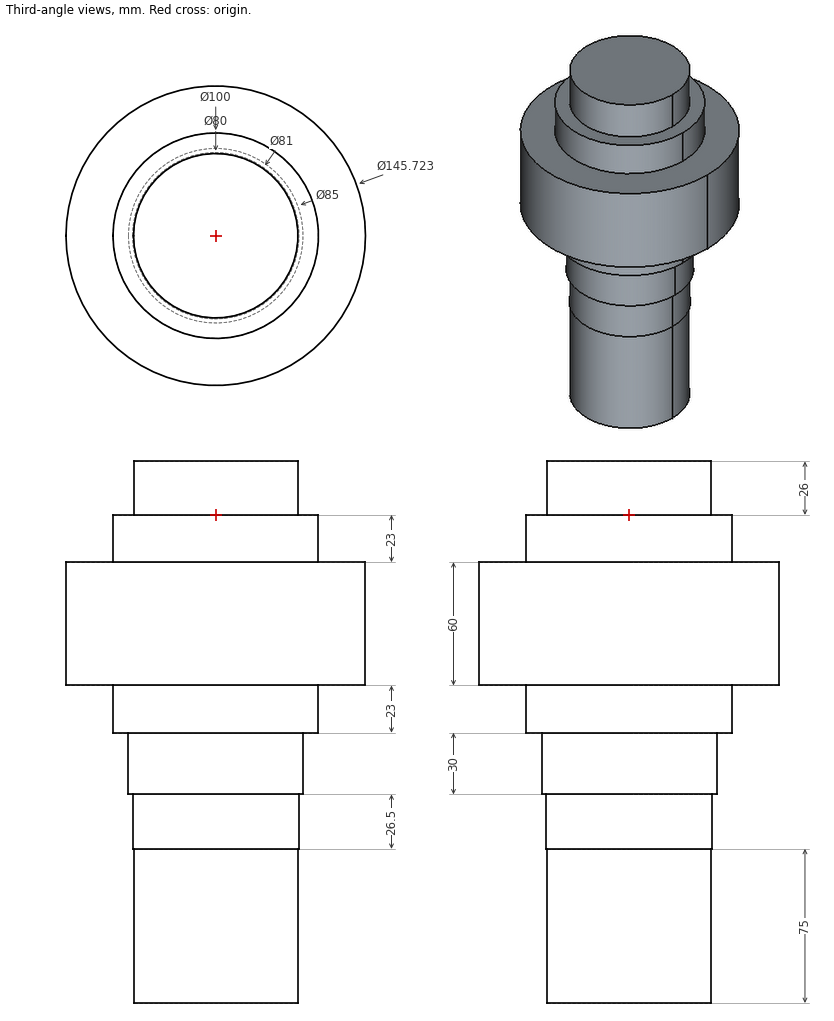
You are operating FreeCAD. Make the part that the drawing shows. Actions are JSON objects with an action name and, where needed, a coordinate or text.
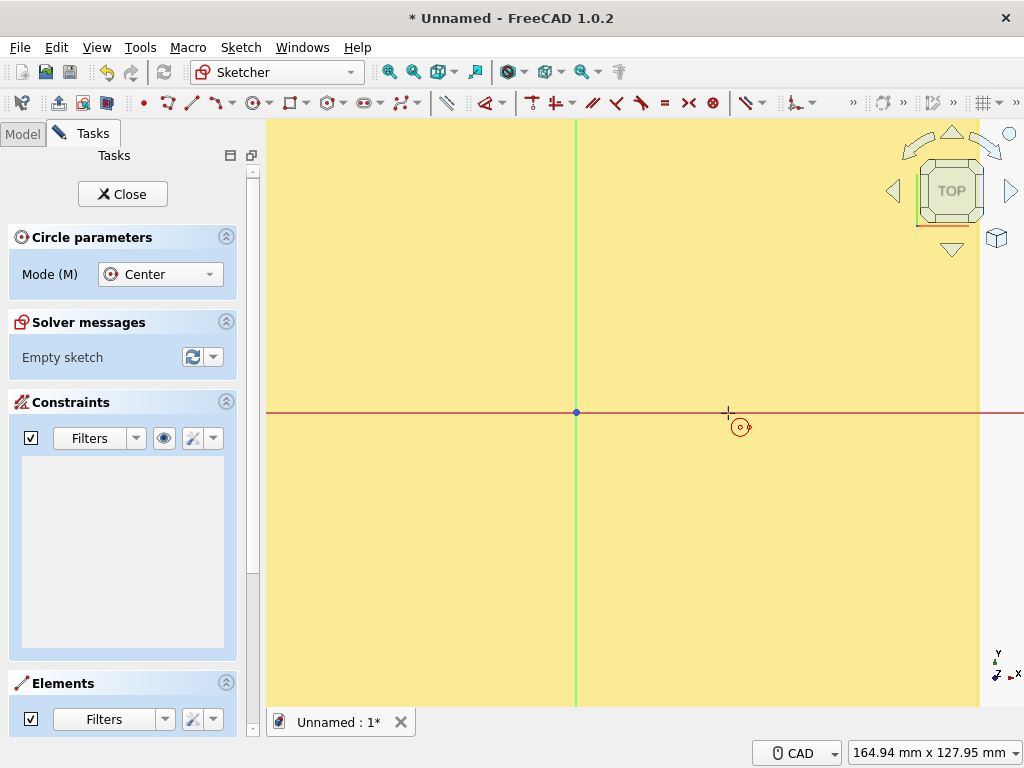
{"action": "left_click", "coordinate": [576, 413]}
{"action": "left_click", "coordinate": [706, 283]}
{"action": "key", "text": "Escape"}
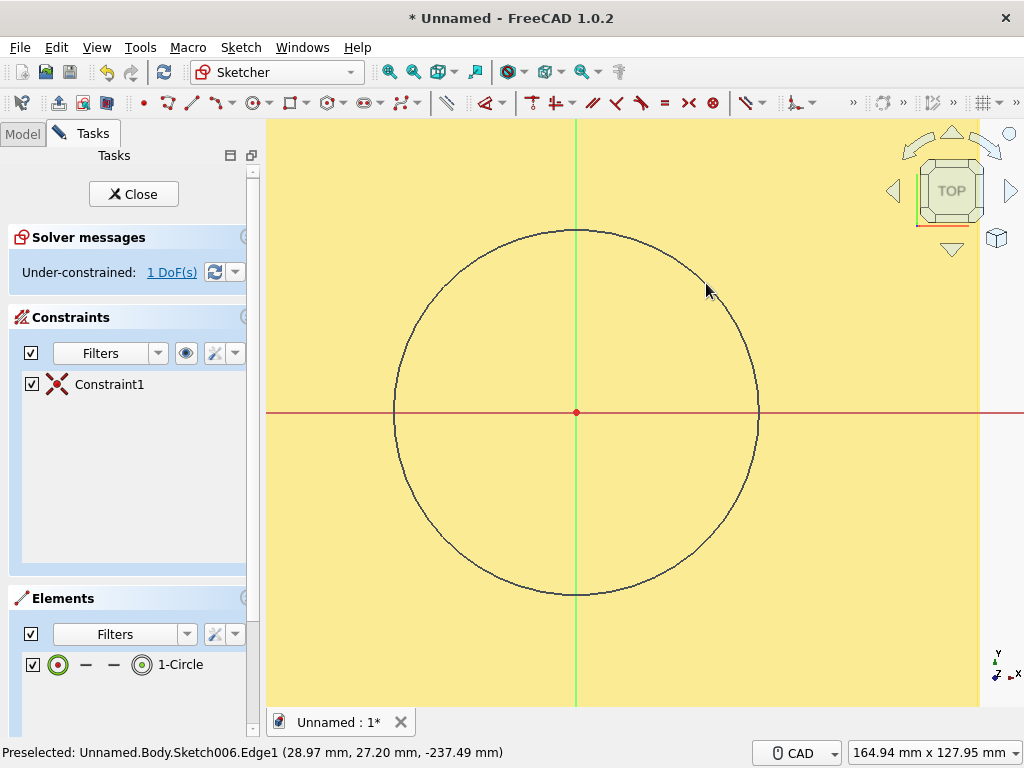
{"action": "key", "text": "d"}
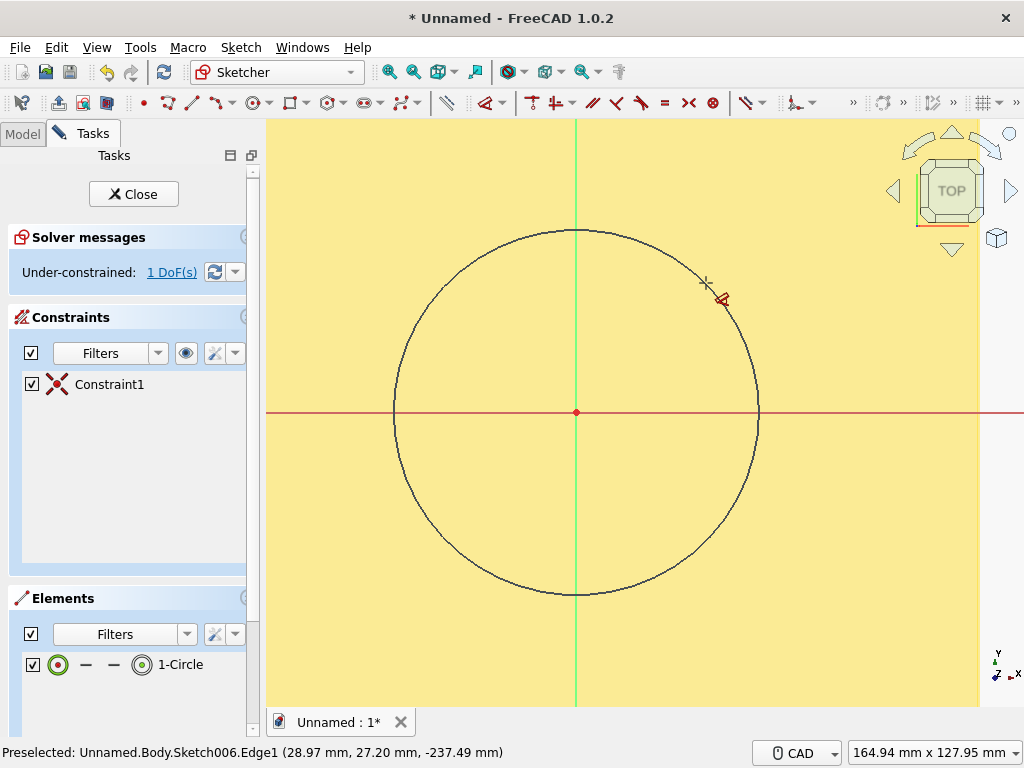
{"action": "left_click", "coordinate": [705, 283]}
{"action": "left_click", "coordinate": [728, 260]}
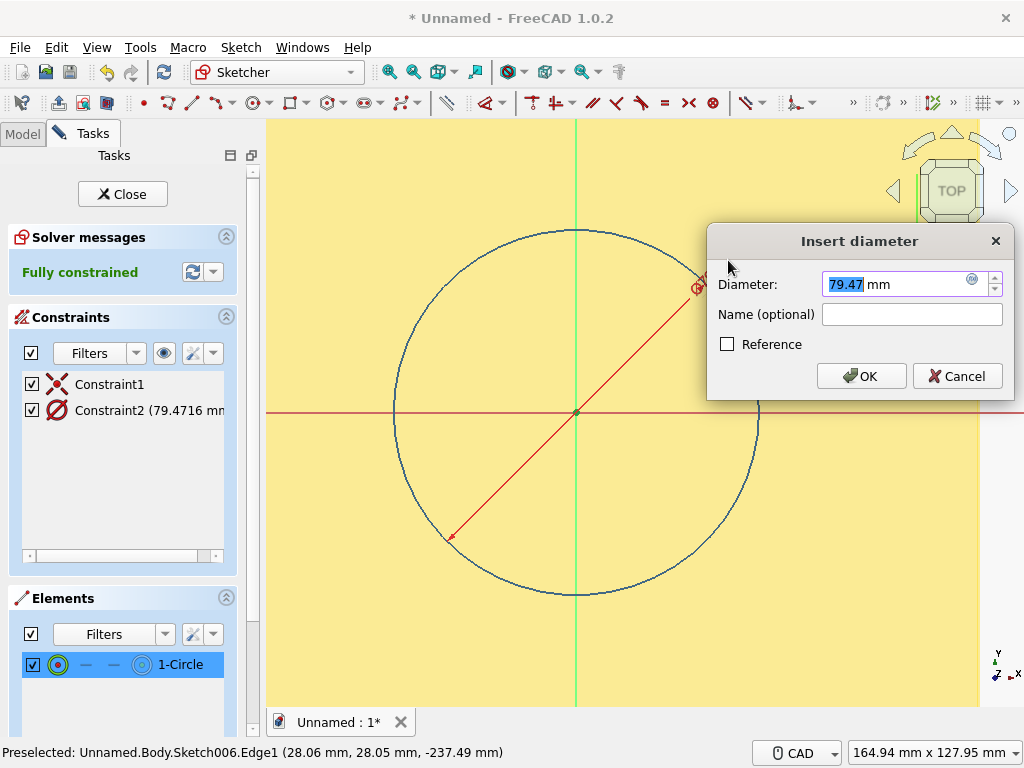
{"action": "type", "text": "80"}
{"action": "key", "text": "Return"}
{"action": "key", "text": "Escape"}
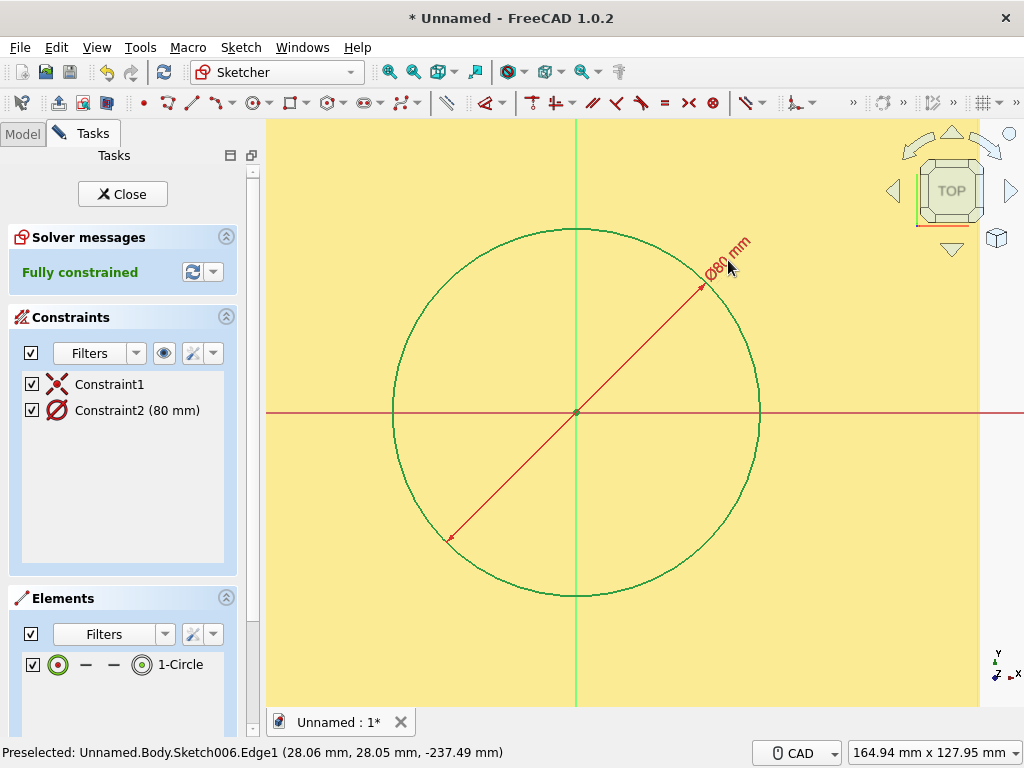
{"action": "left_click", "coordinate": [123, 194]}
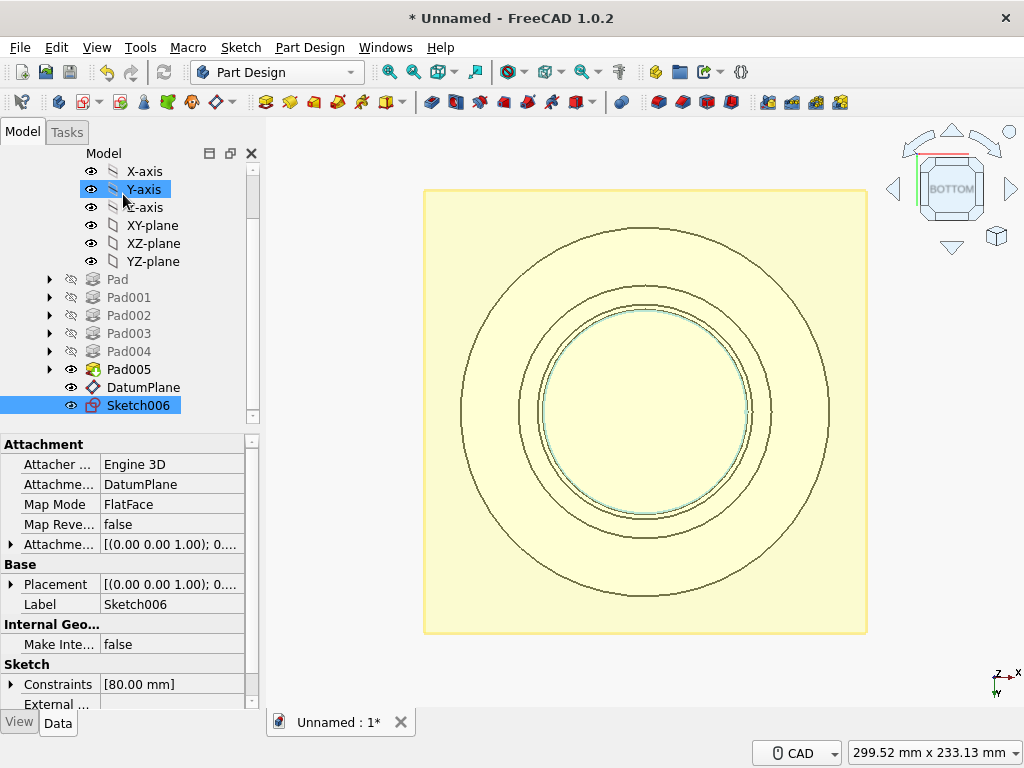
{"action": "left_click", "coordinate": [266, 102]}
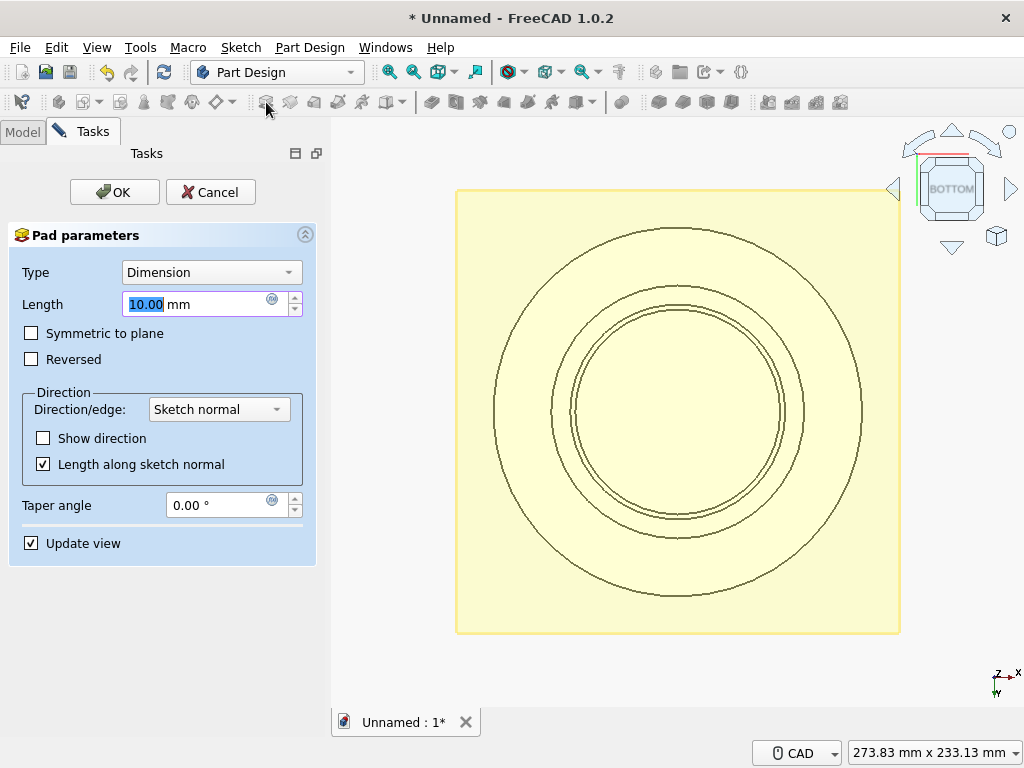
{"action": "type", "text": "75"}
{"action": "key", "text": "Tab"}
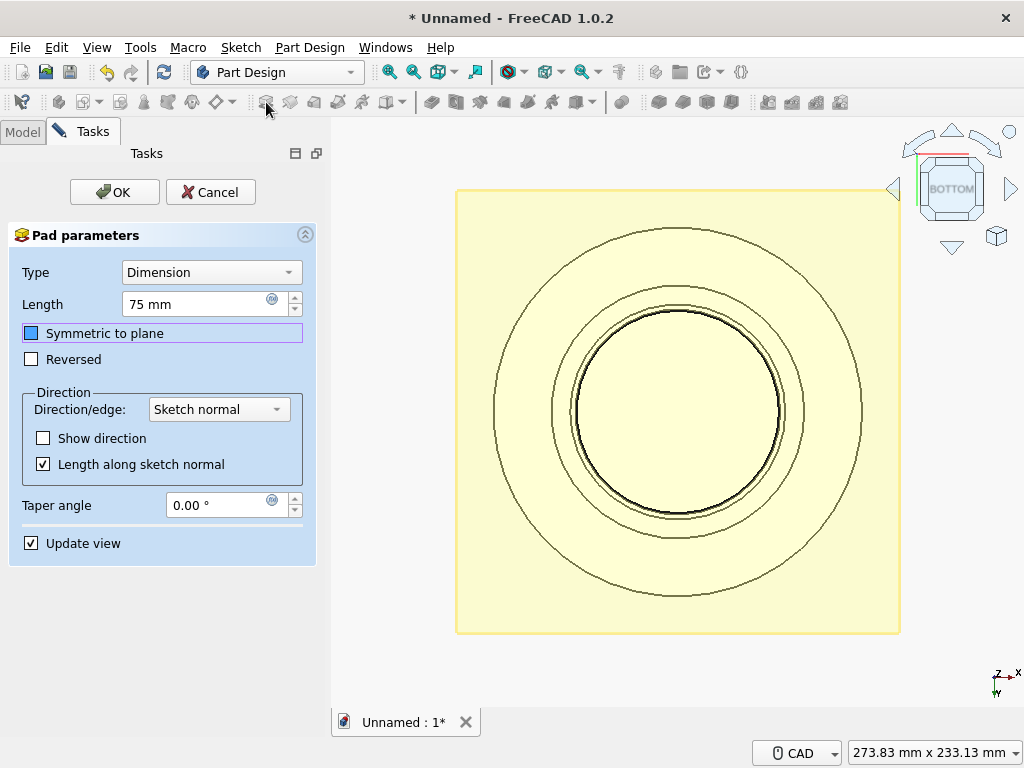
{"action": "left_click", "coordinate": [115, 192]}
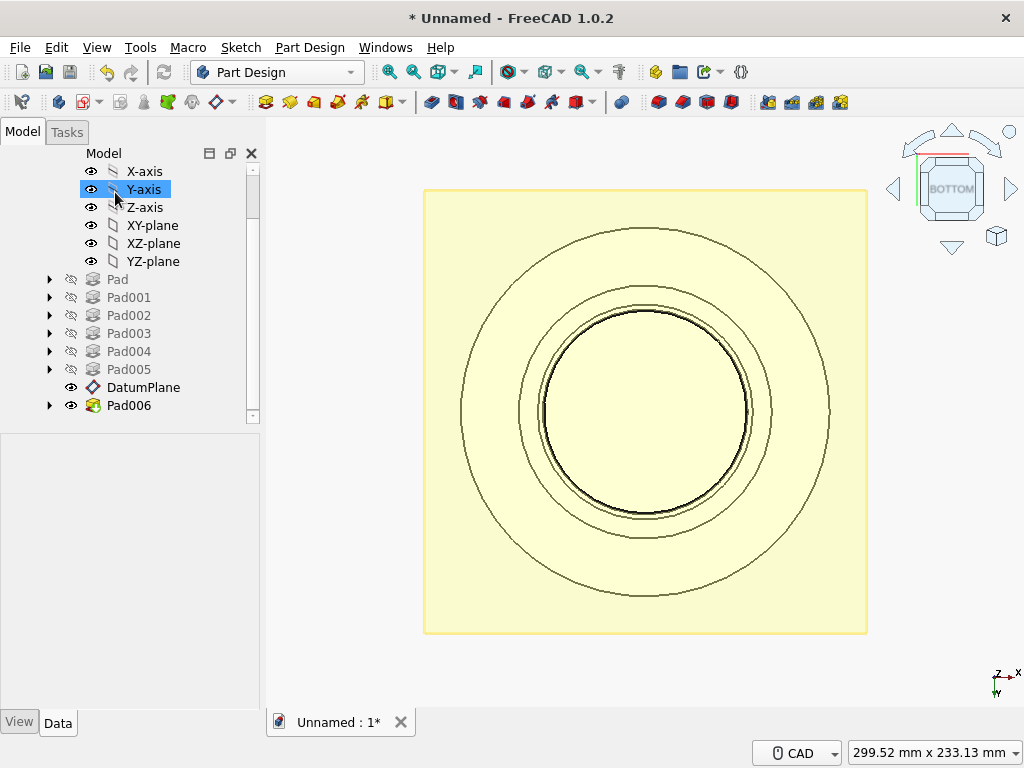
{"action": "left_click", "coordinate": [116, 387]}
{"action": "key", "text": "space"}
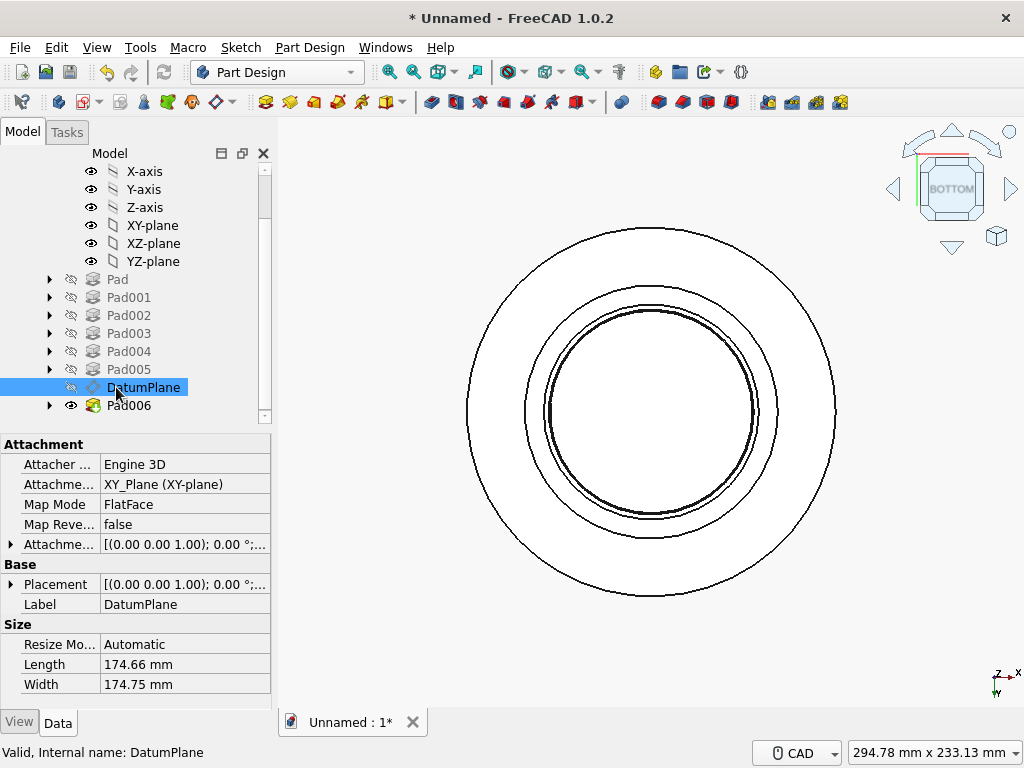
{"action": "key", "text": "0"}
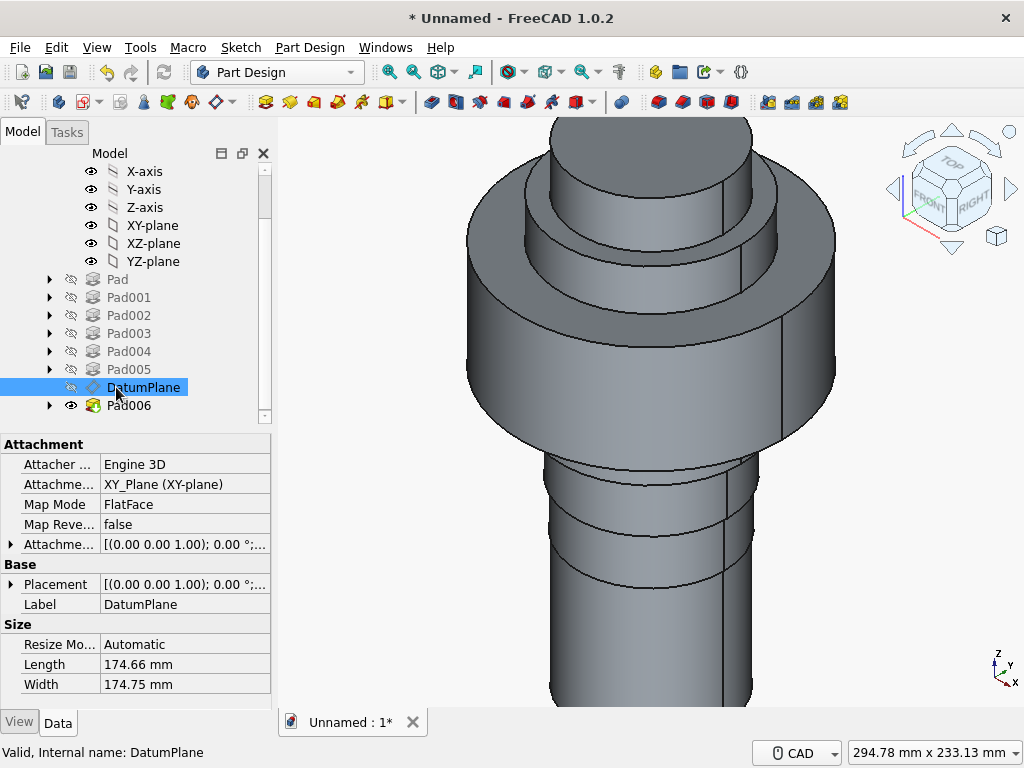
{"action": "left_click", "coordinate": [390, 72]}